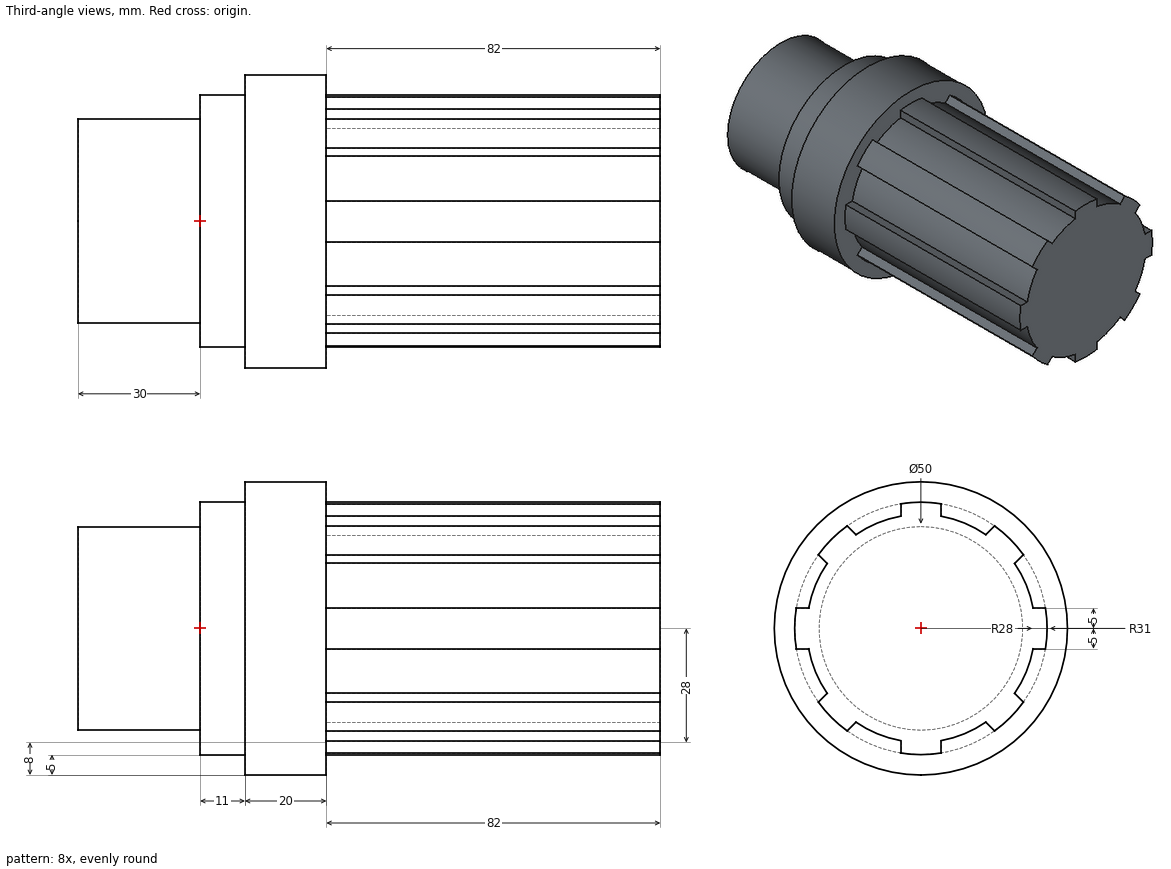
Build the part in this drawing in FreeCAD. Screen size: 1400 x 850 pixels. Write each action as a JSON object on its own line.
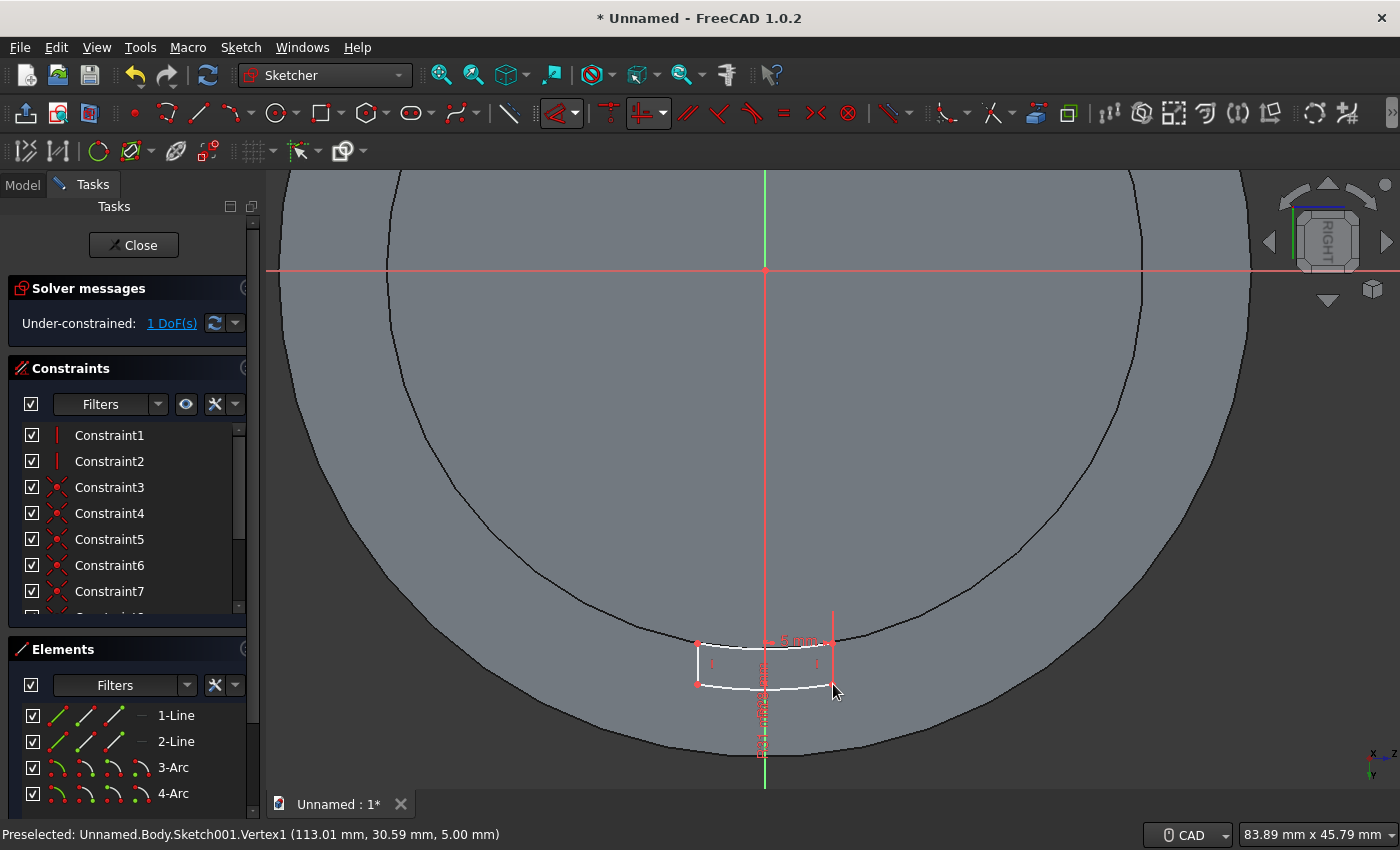
{"action": "left_click", "coordinate": [698, 643]}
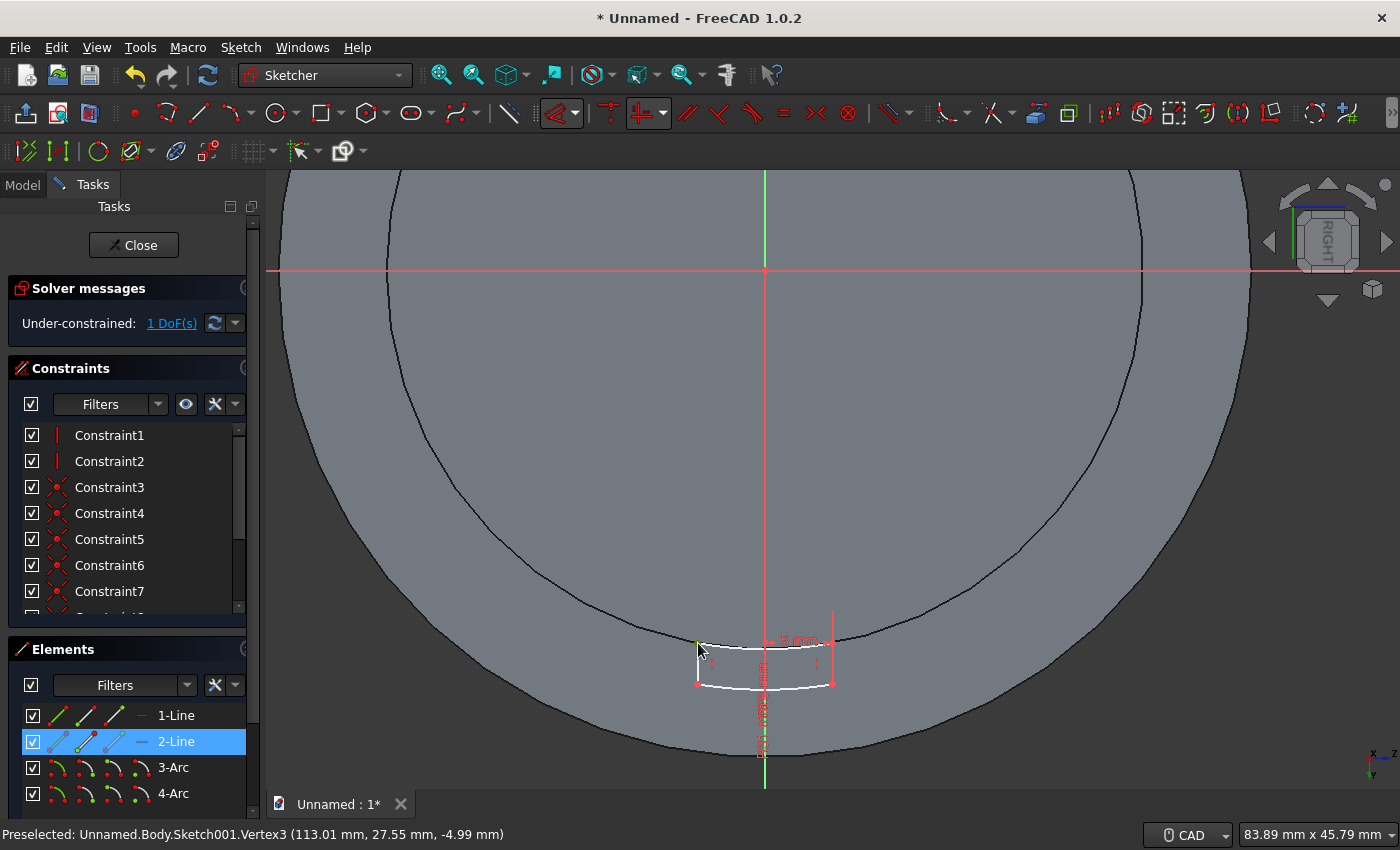
{"action": "left_click", "coordinate": [578, 114]}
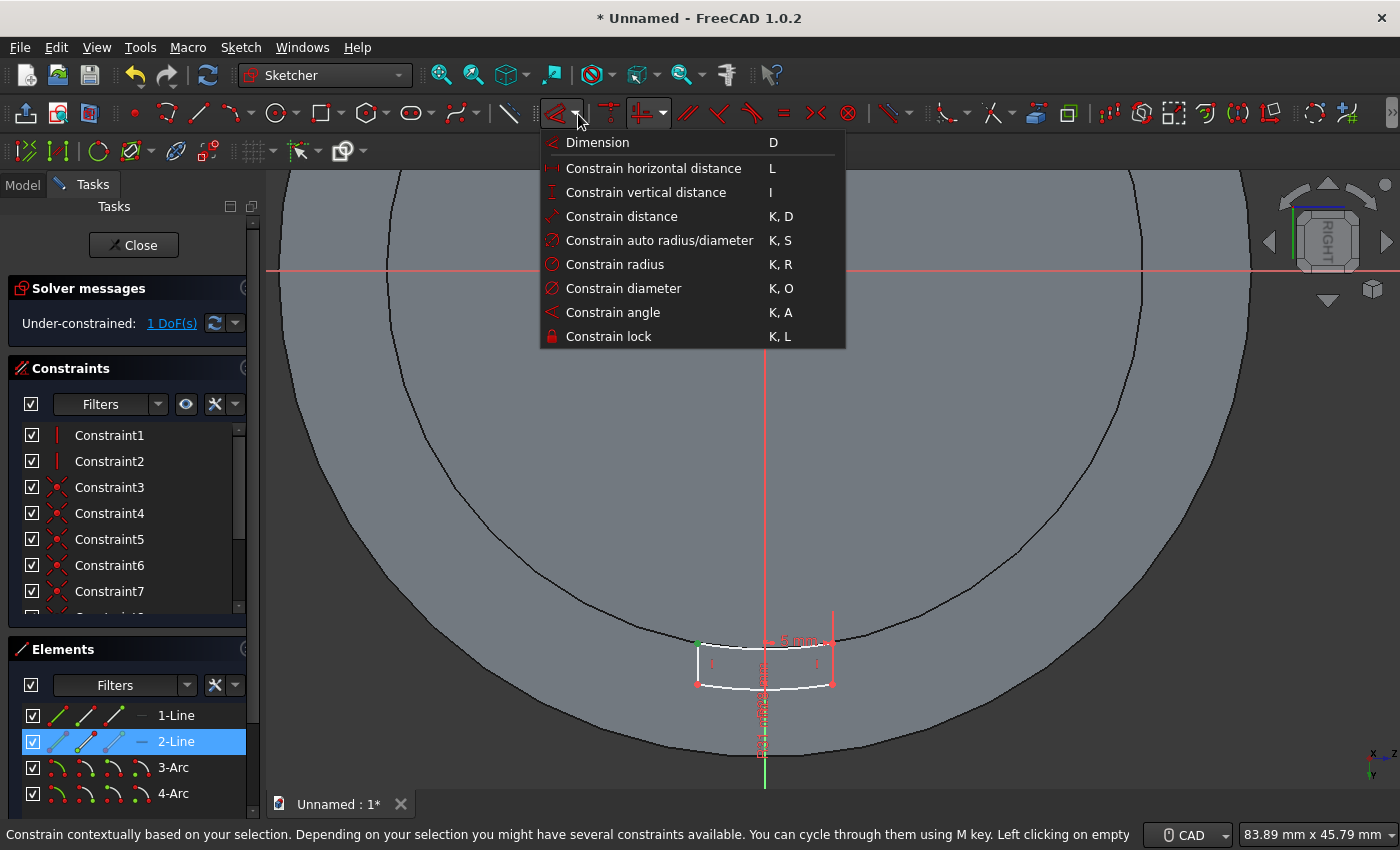
{"action": "left_click", "coordinate": [693, 168]}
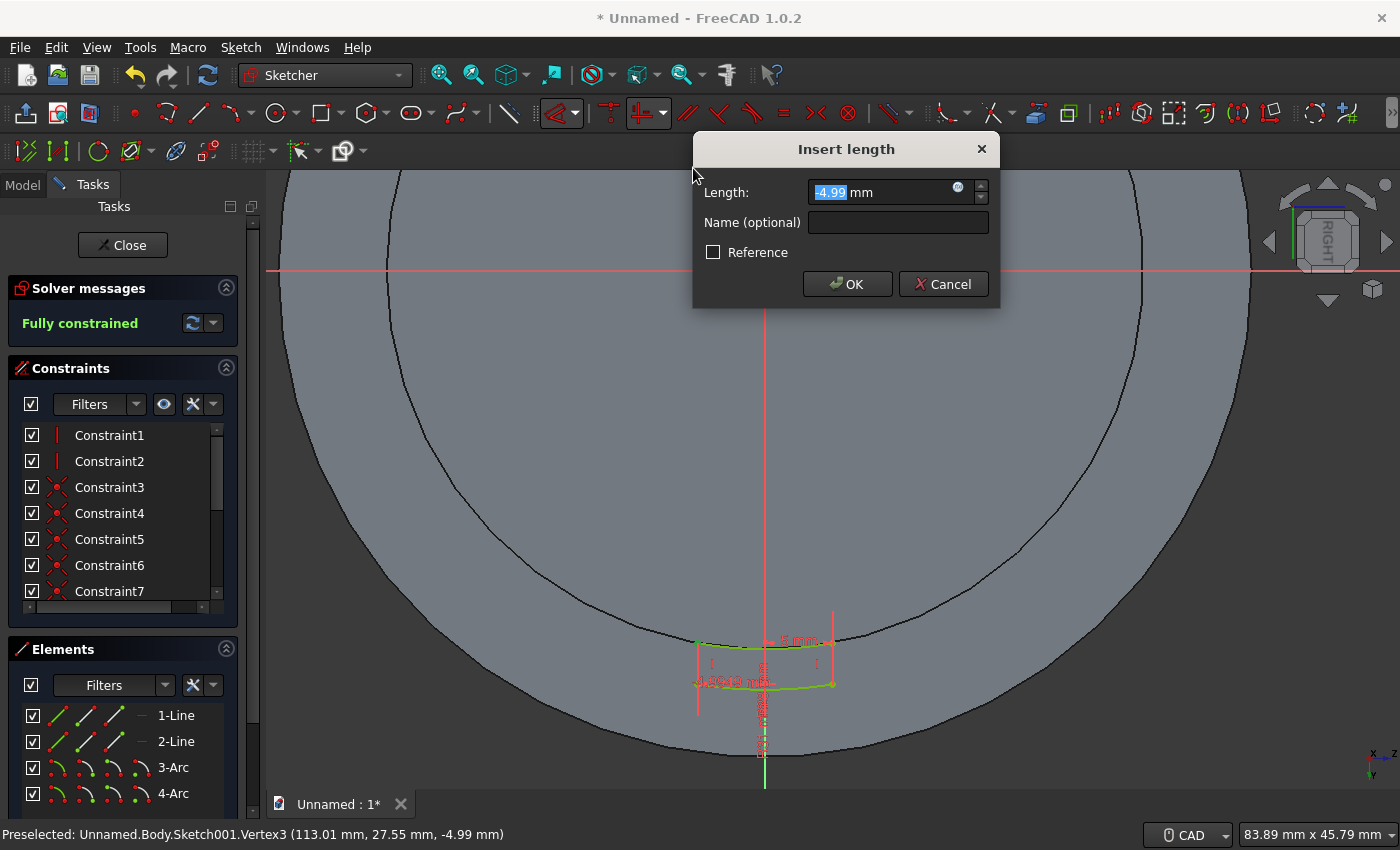
{"action": "type", "text": "-5"}
{"action": "key", "text": "Return"}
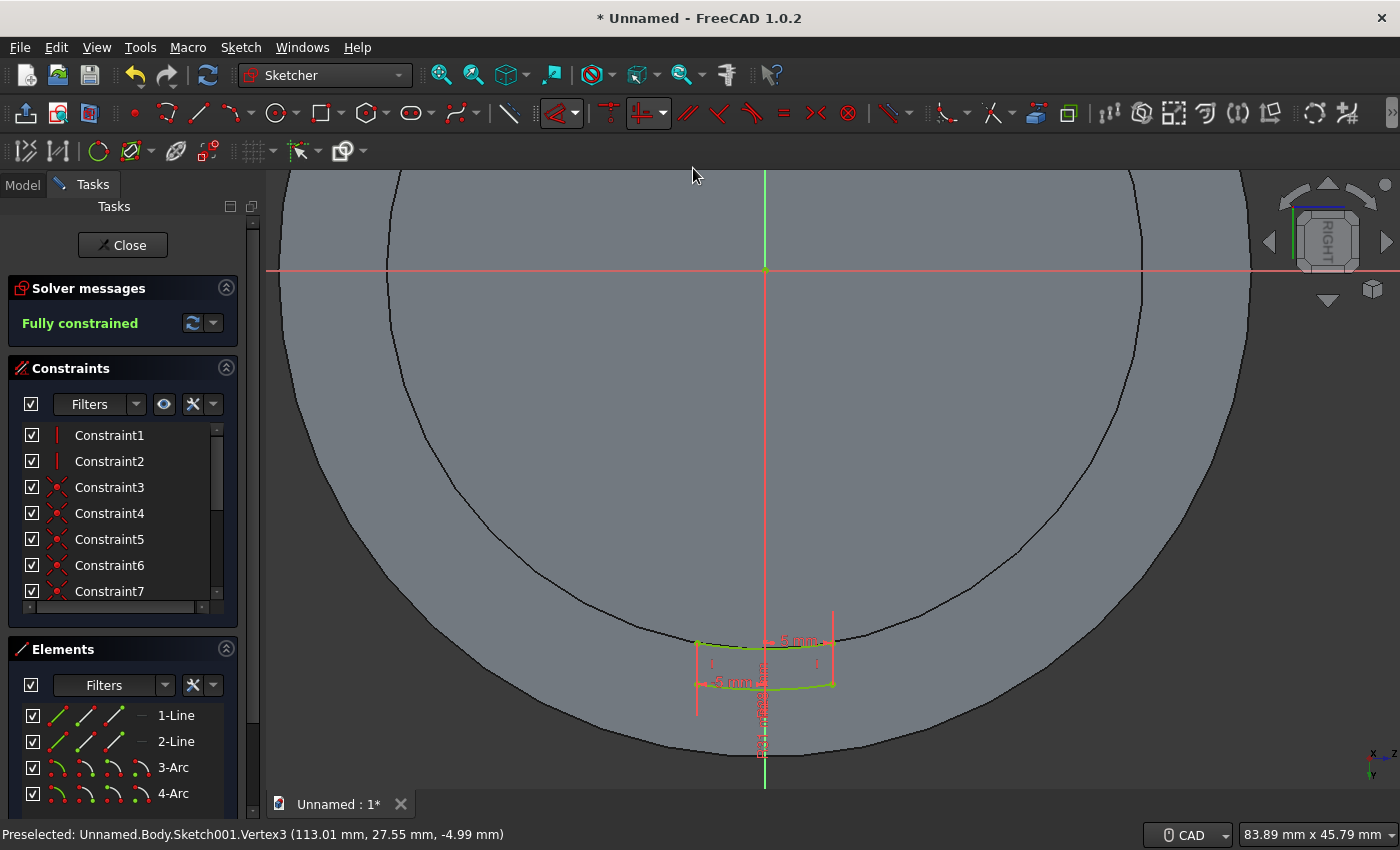
{"action": "left_click", "coordinate": [123, 245]}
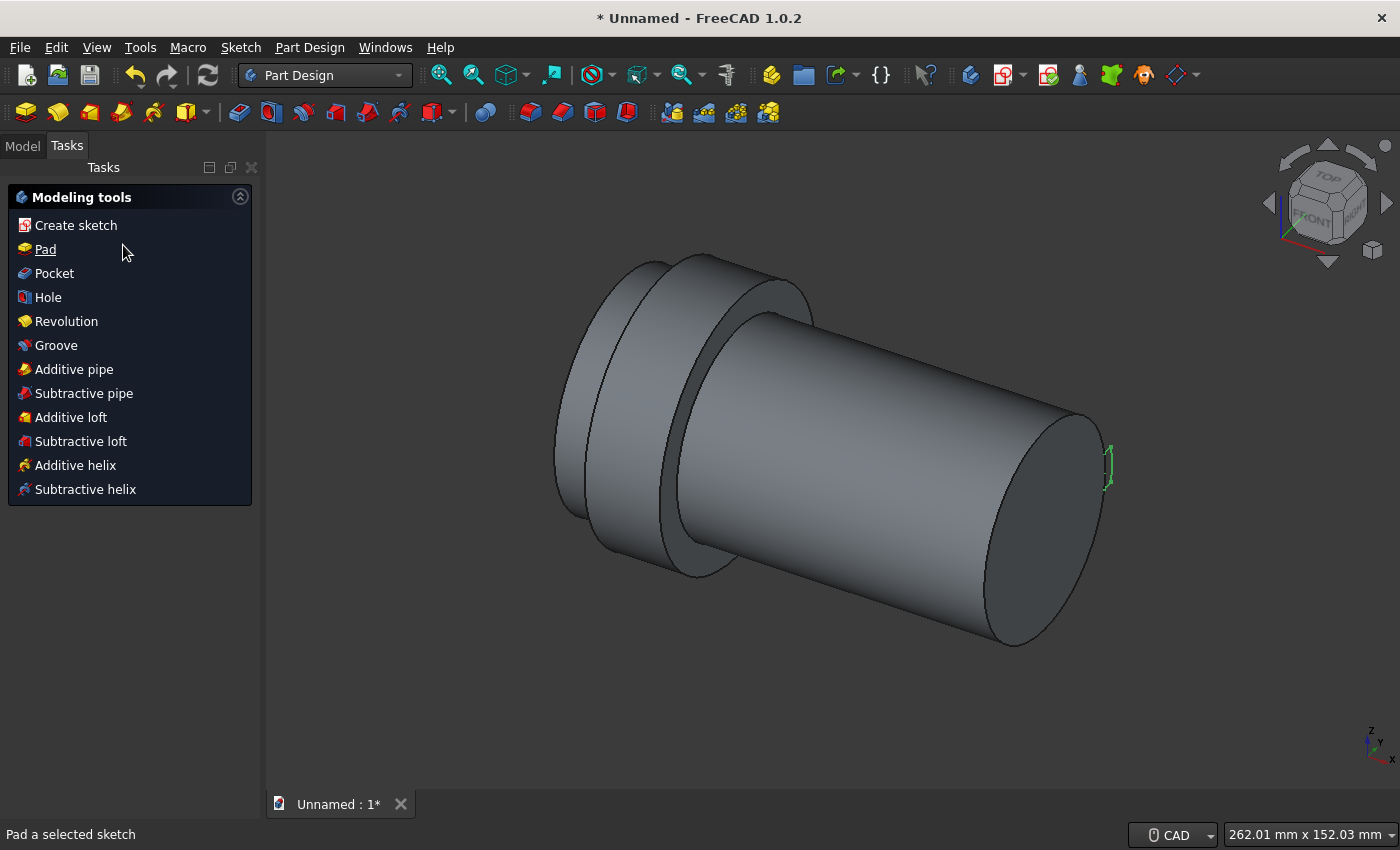
{"action": "left_click", "coordinate": [26, 112]}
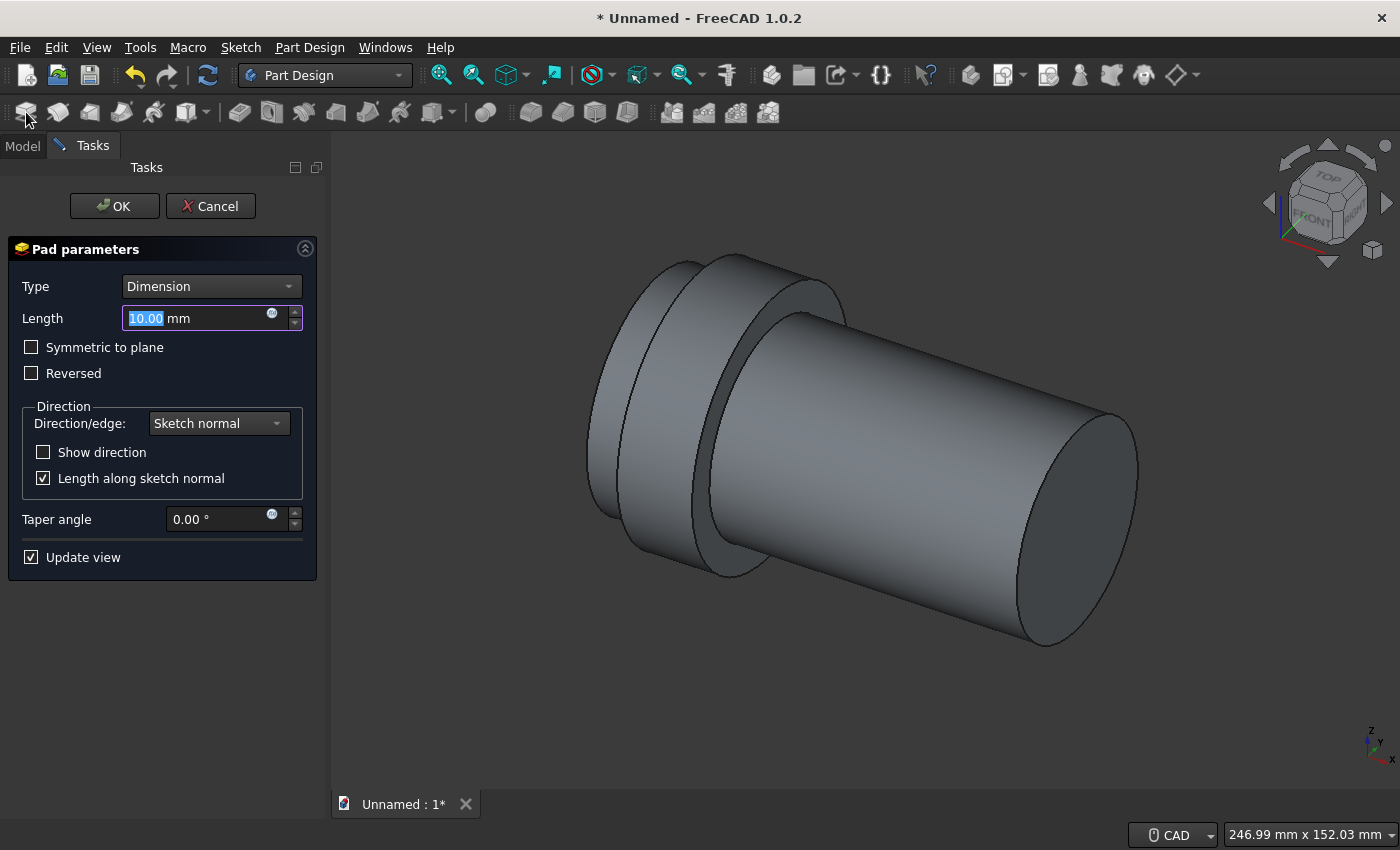
{"action": "type", "text": "82"}
{"action": "key", "text": "Tab"}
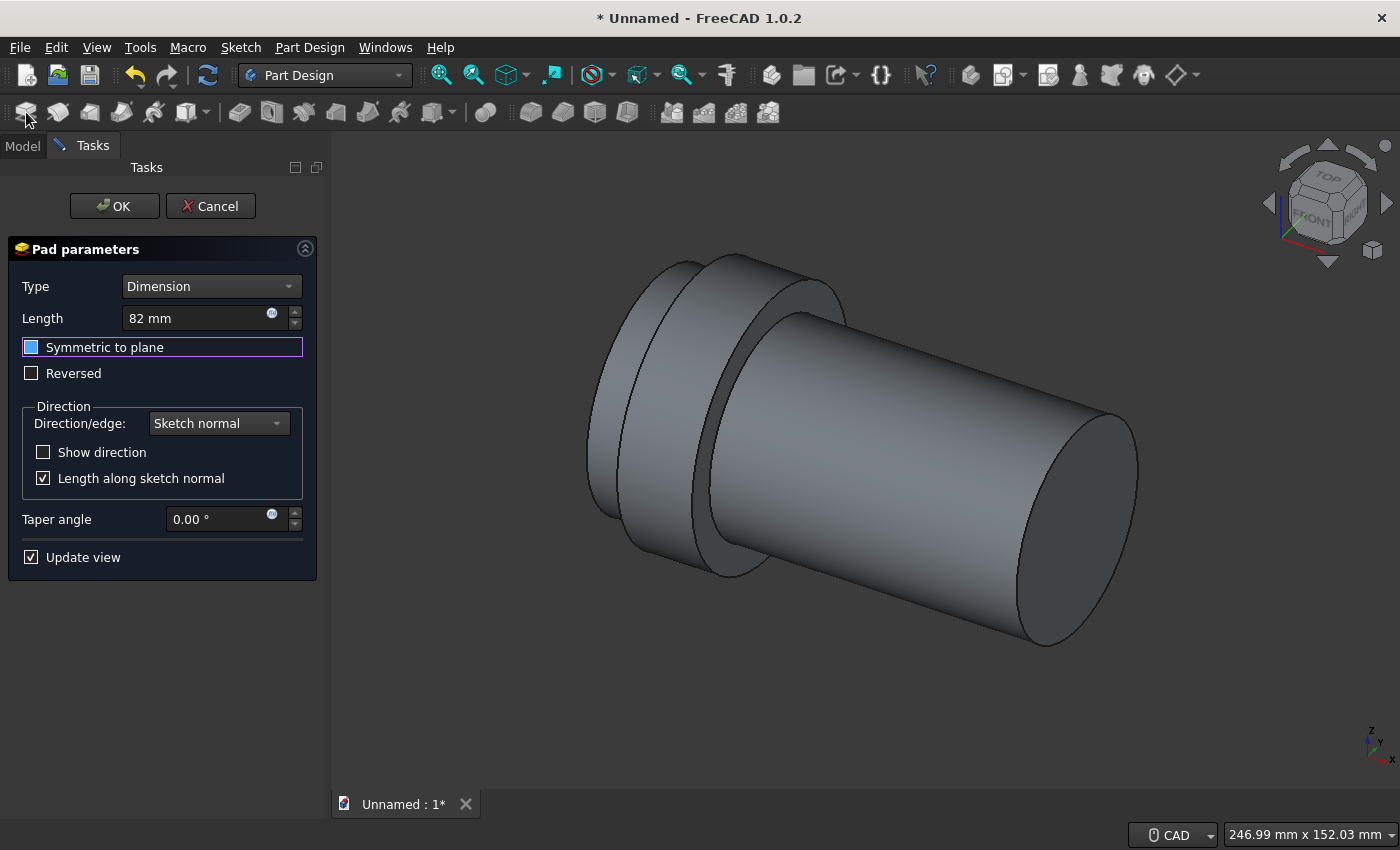
{"action": "left_click", "coordinate": [30, 373]}